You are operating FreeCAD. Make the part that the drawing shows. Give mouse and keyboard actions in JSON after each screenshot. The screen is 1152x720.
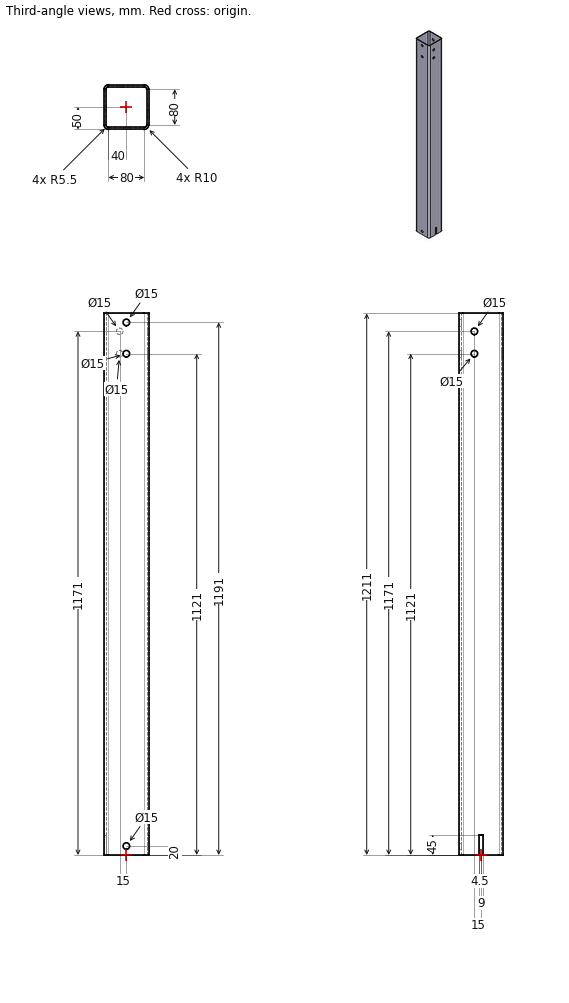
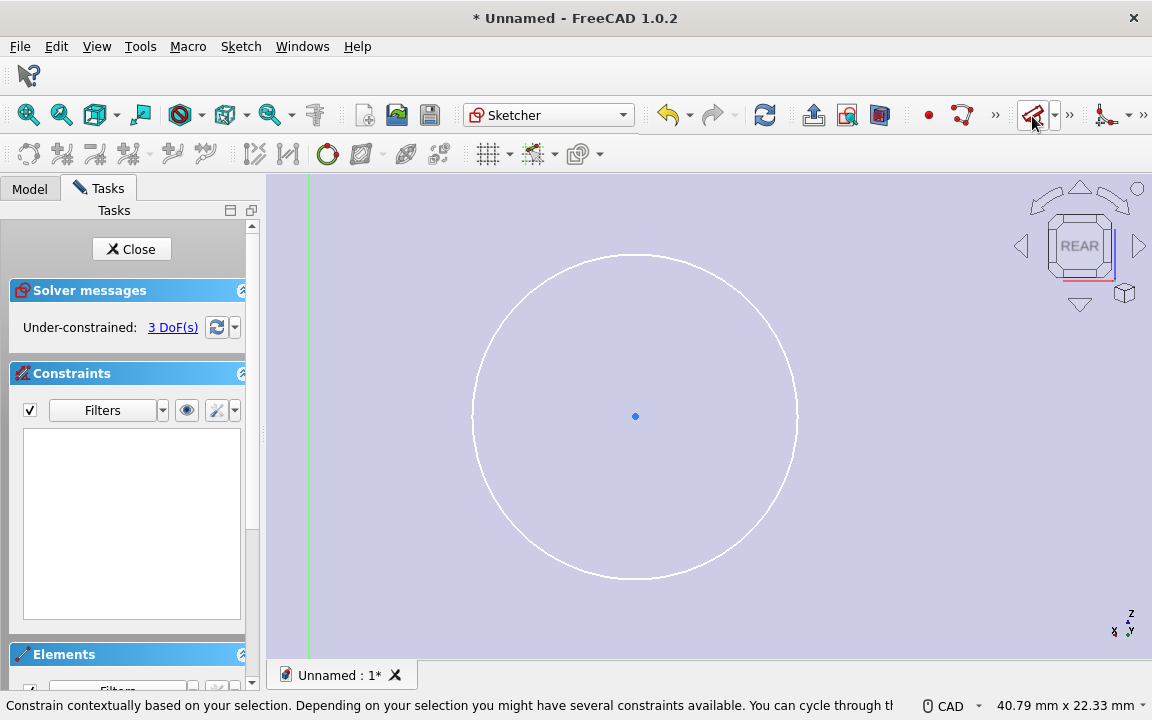
{"action": "left_click", "coordinate": [750, 302]}
{"action": "left_click", "coordinate": [773, 279]}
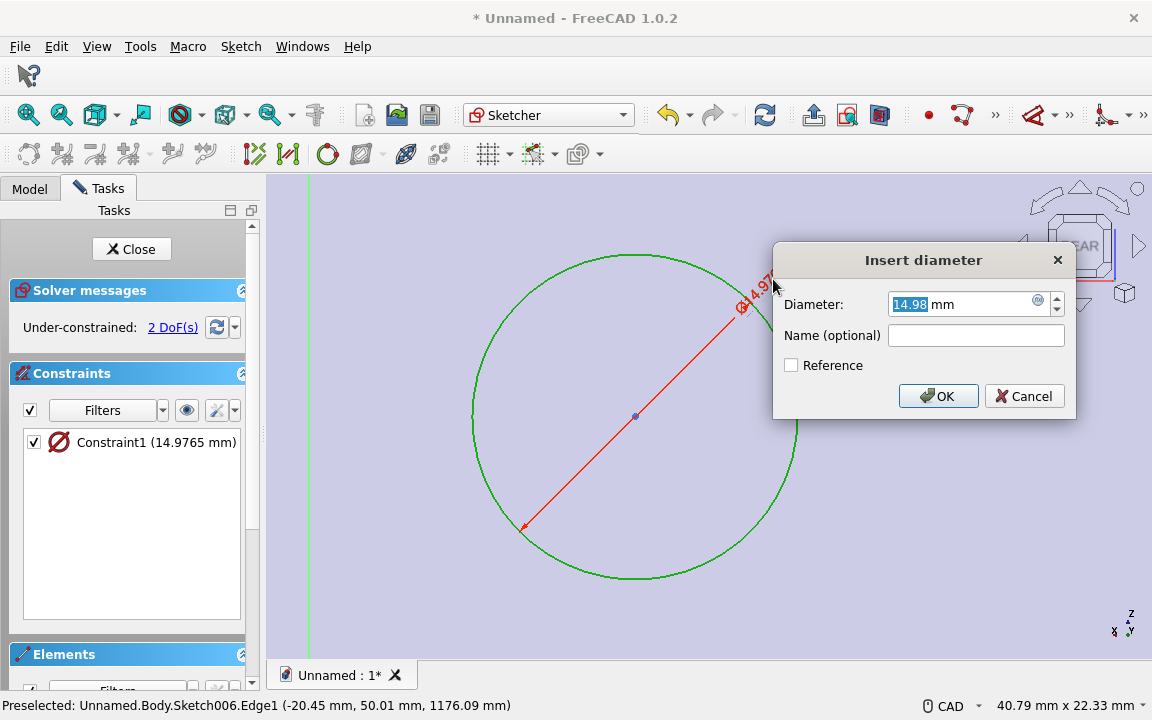
{"action": "type", "text": "15"}
{"action": "key", "text": "Return"}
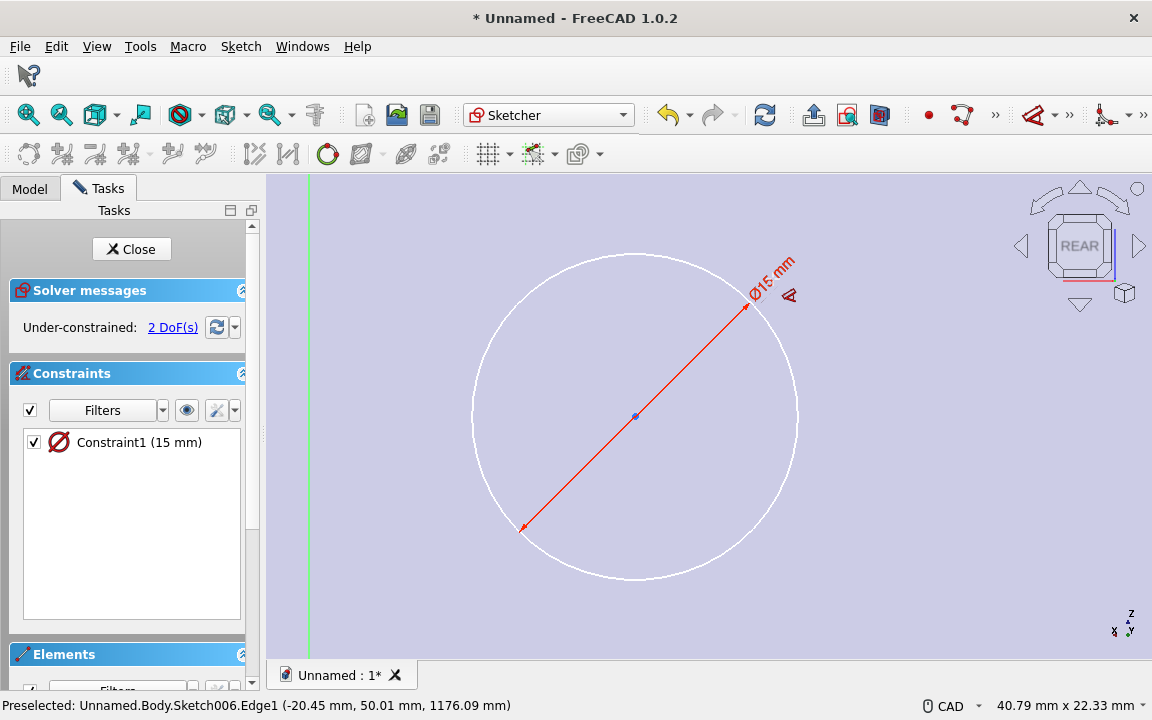
{"action": "left_click", "coordinate": [635, 417]}
{"action": "left_click", "coordinate": [397, 383]}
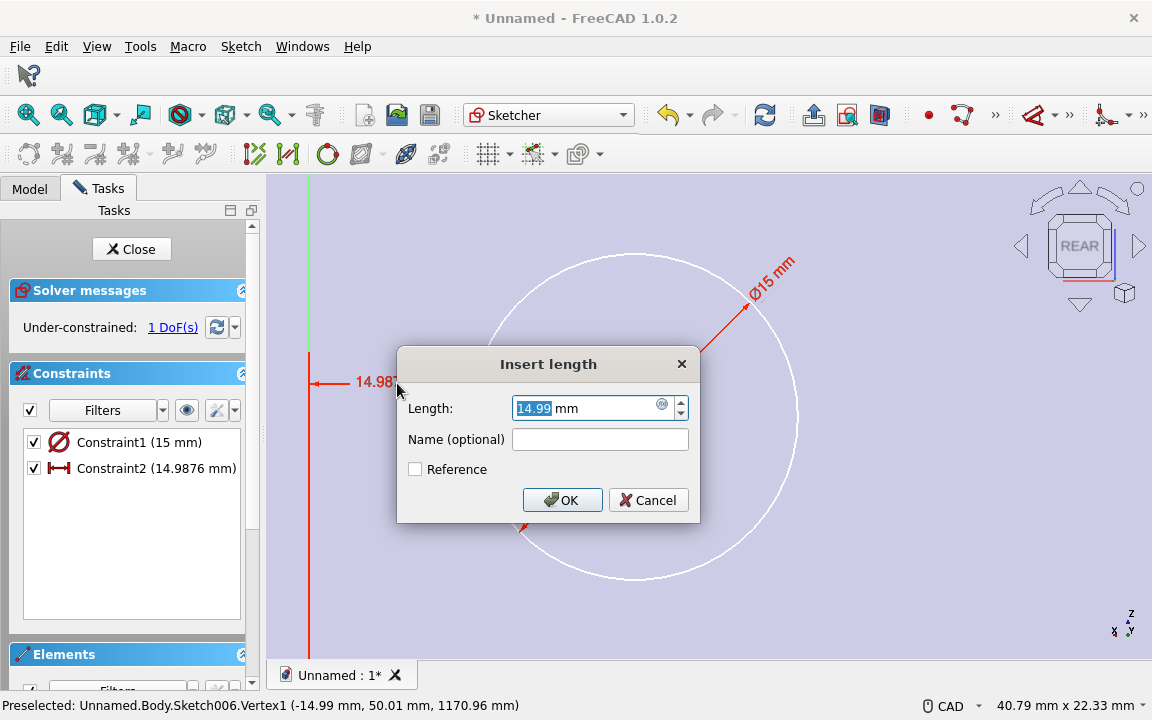
{"action": "type", "text": "15"}
{"action": "key", "text": "Return"}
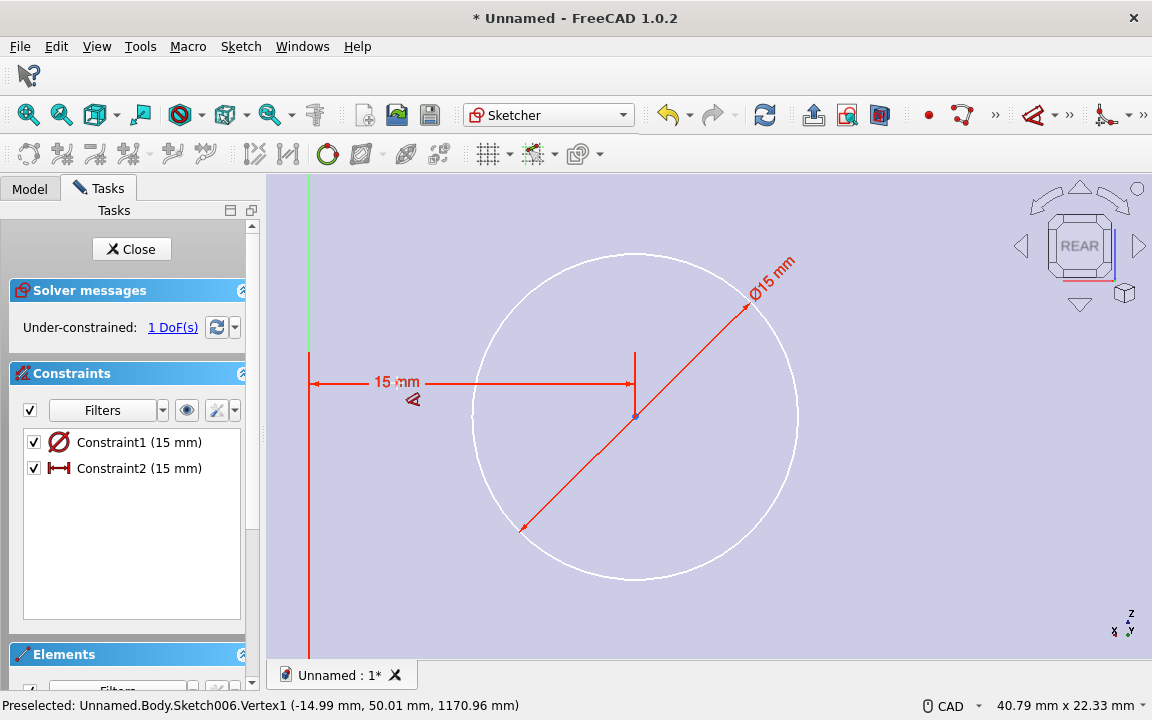
{"action": "left_click", "coordinate": [635, 417]}
{"action": "left_click", "coordinate": [669, 524]}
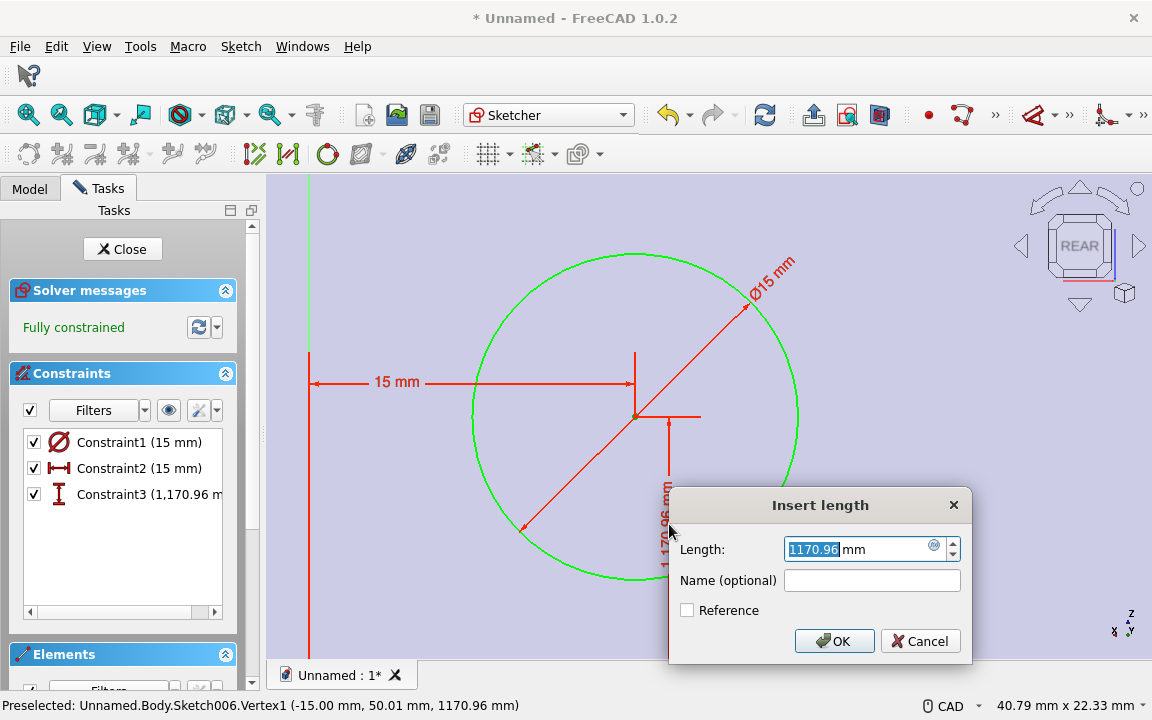
{"action": "type", "text": "1171"}
{"action": "key", "text": "Return"}
{"action": "key", "text": "Escape"}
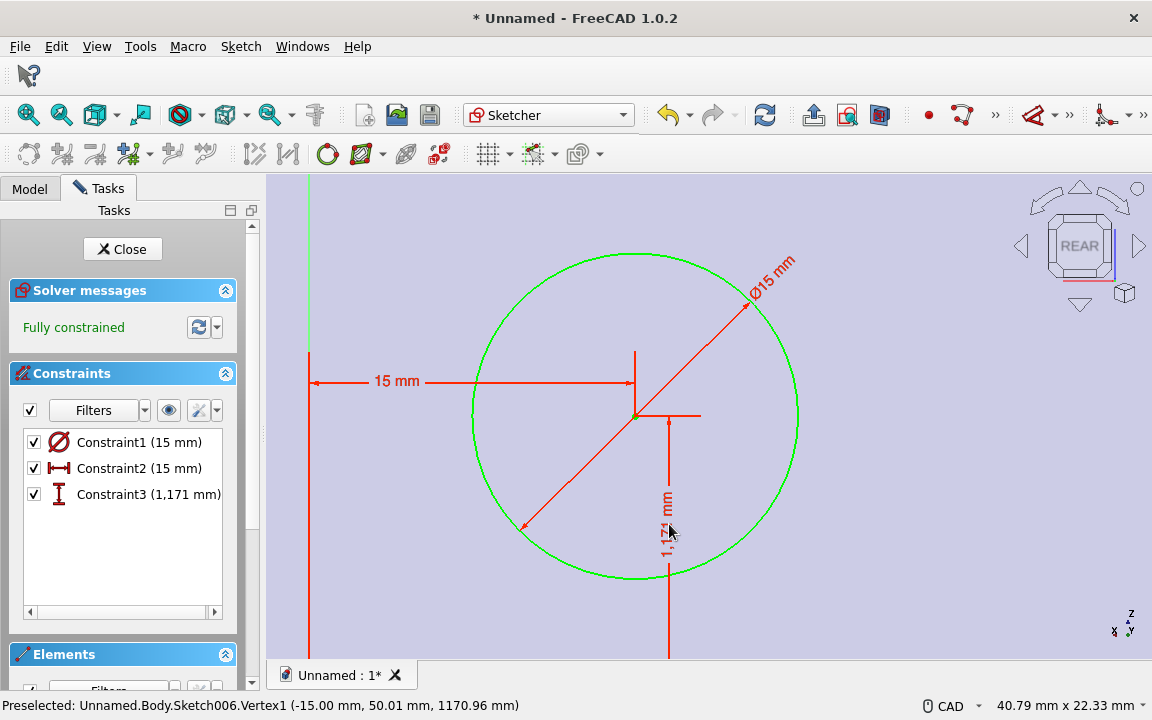
{"action": "left_click", "coordinate": [123, 249]}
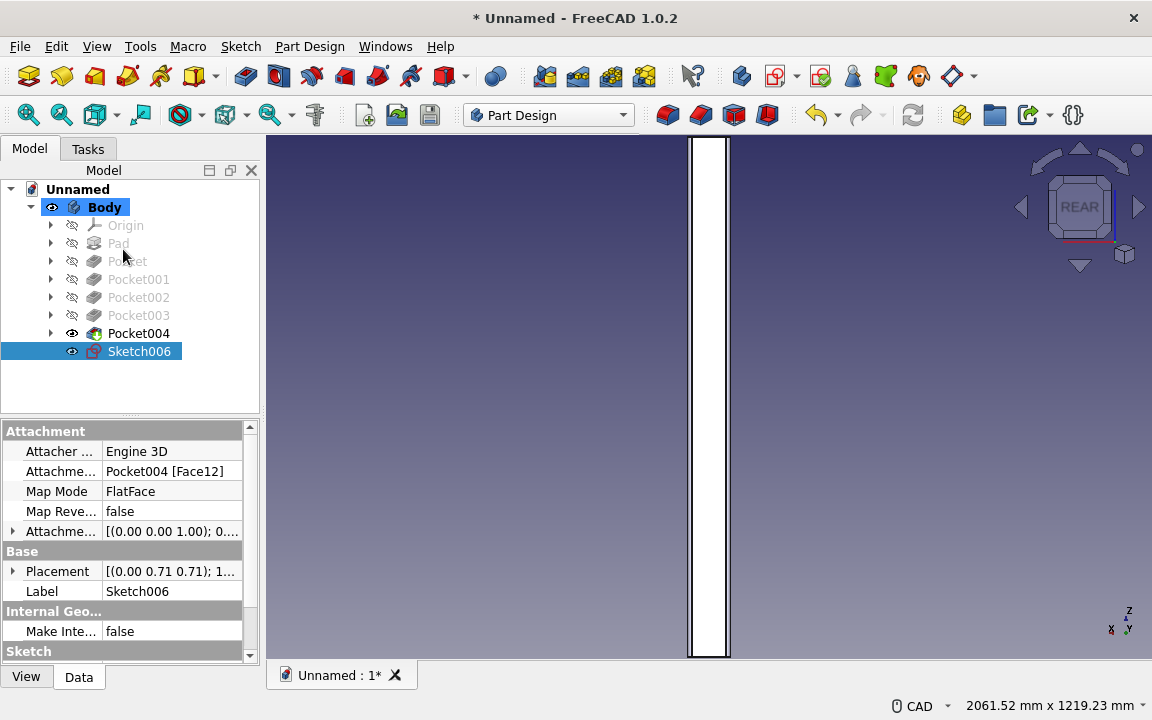
{"action": "left_click", "coordinate": [246, 76]}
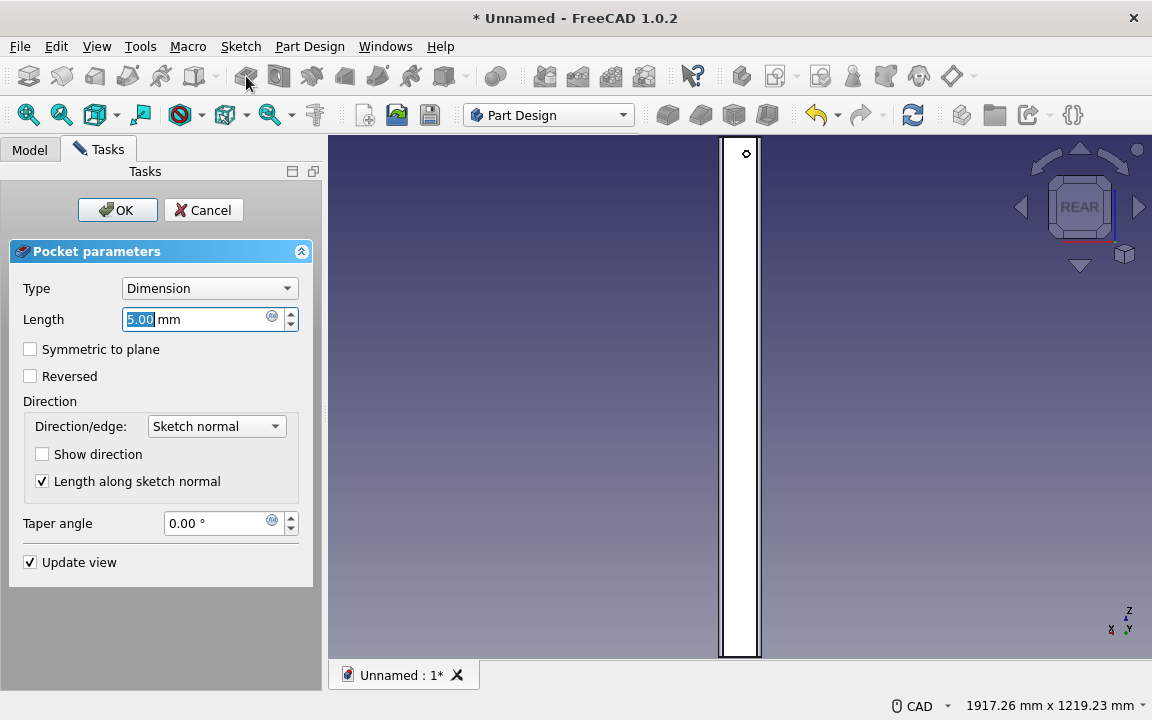
{"action": "left_click", "coordinate": [210, 288]}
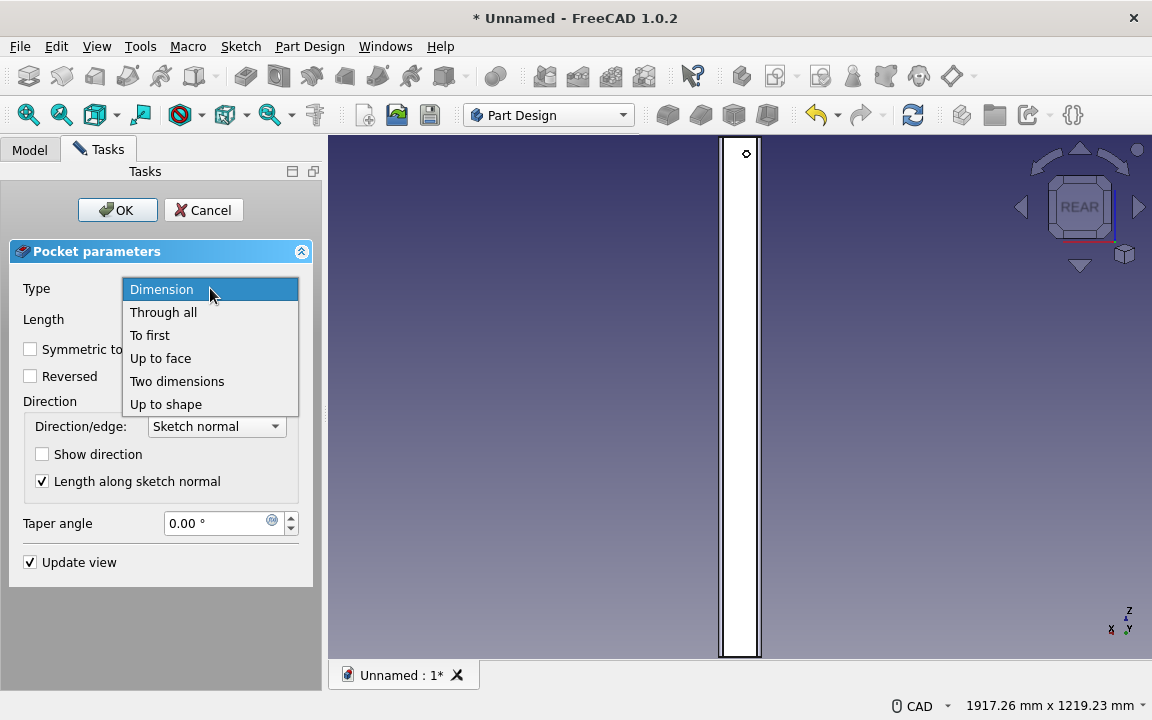
{"action": "left_click", "coordinate": [208, 336]}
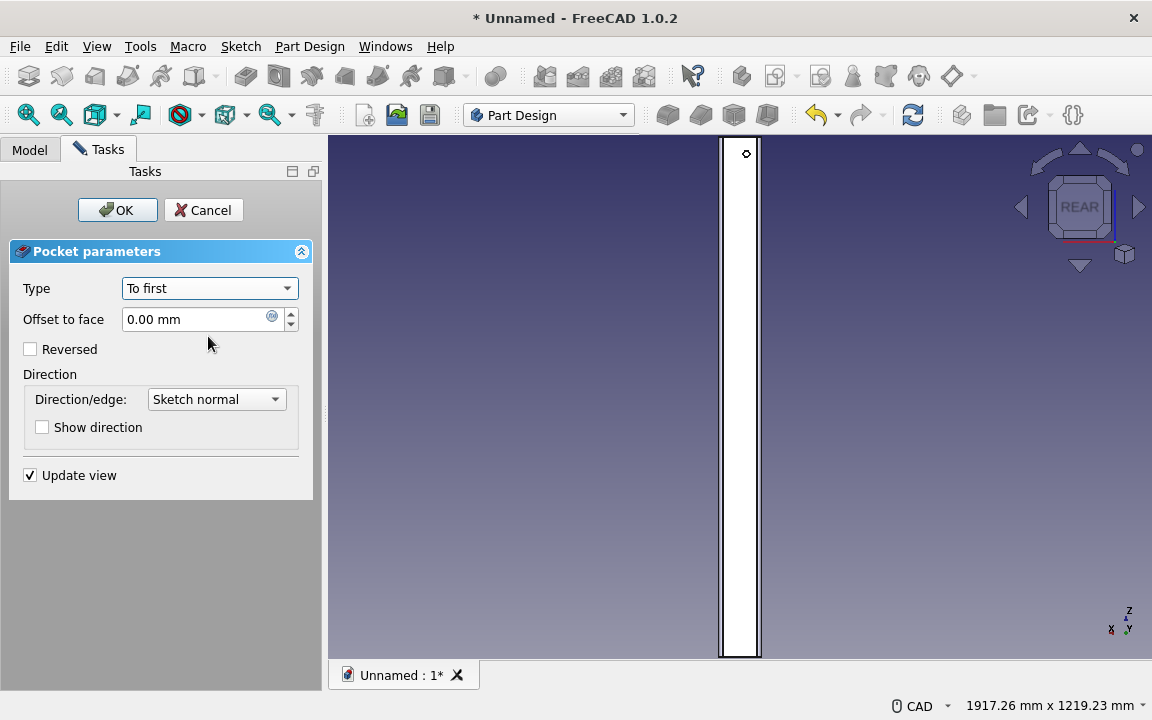
{"action": "left_click", "coordinate": [118, 210]}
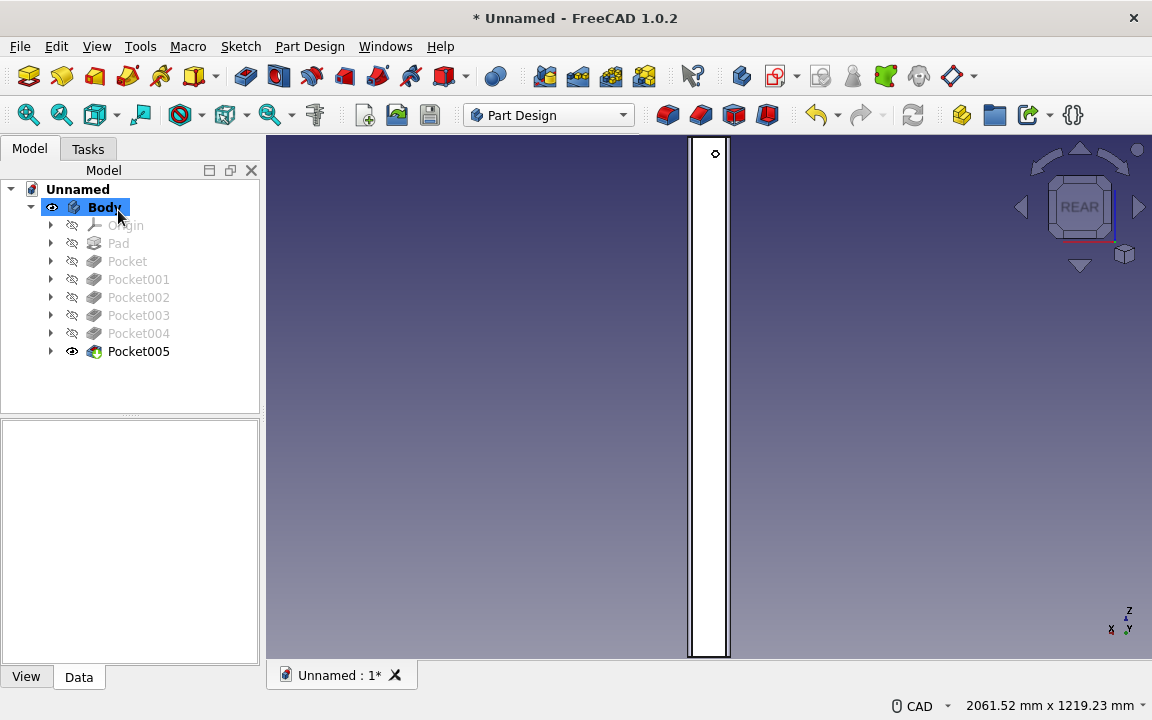
{"action": "left_click", "coordinate": [709, 173]}